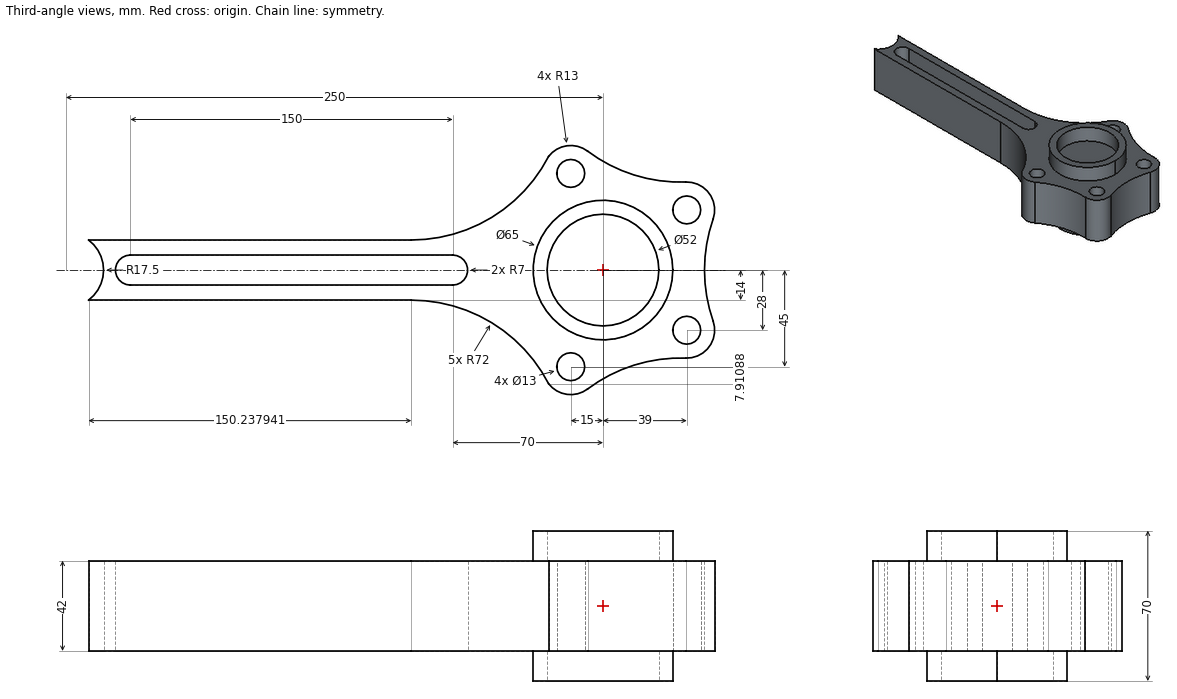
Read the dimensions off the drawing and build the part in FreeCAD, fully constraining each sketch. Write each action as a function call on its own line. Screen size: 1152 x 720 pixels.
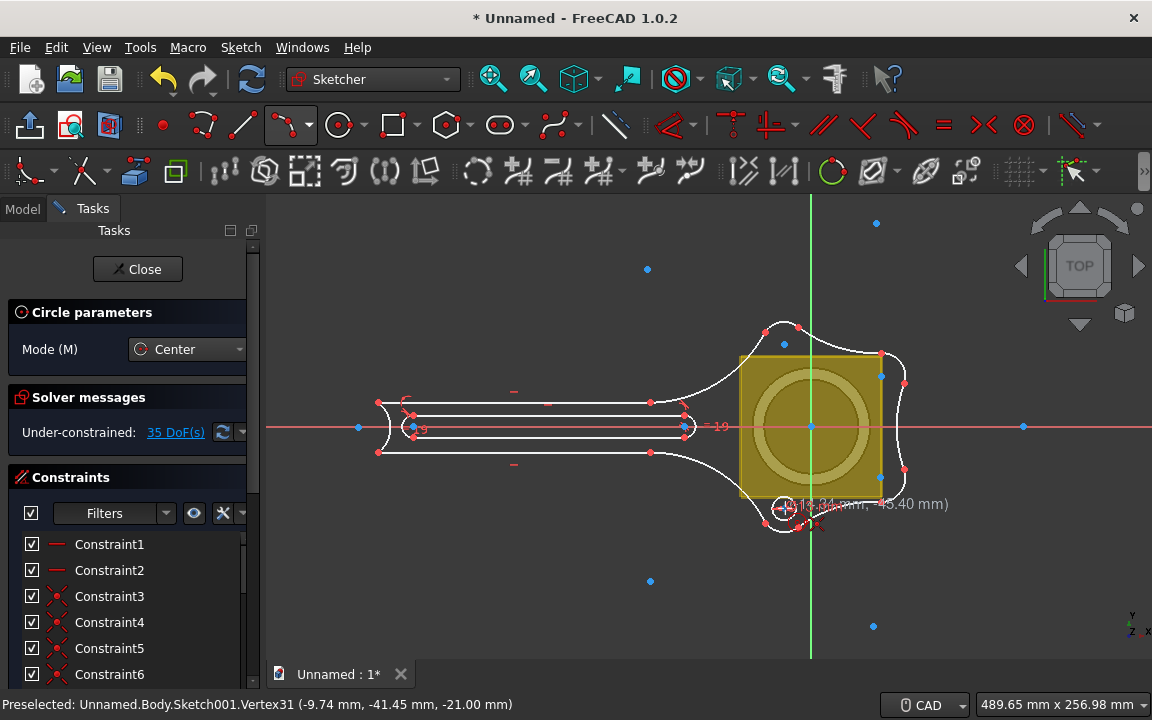
scroll(882, 477, up, 4)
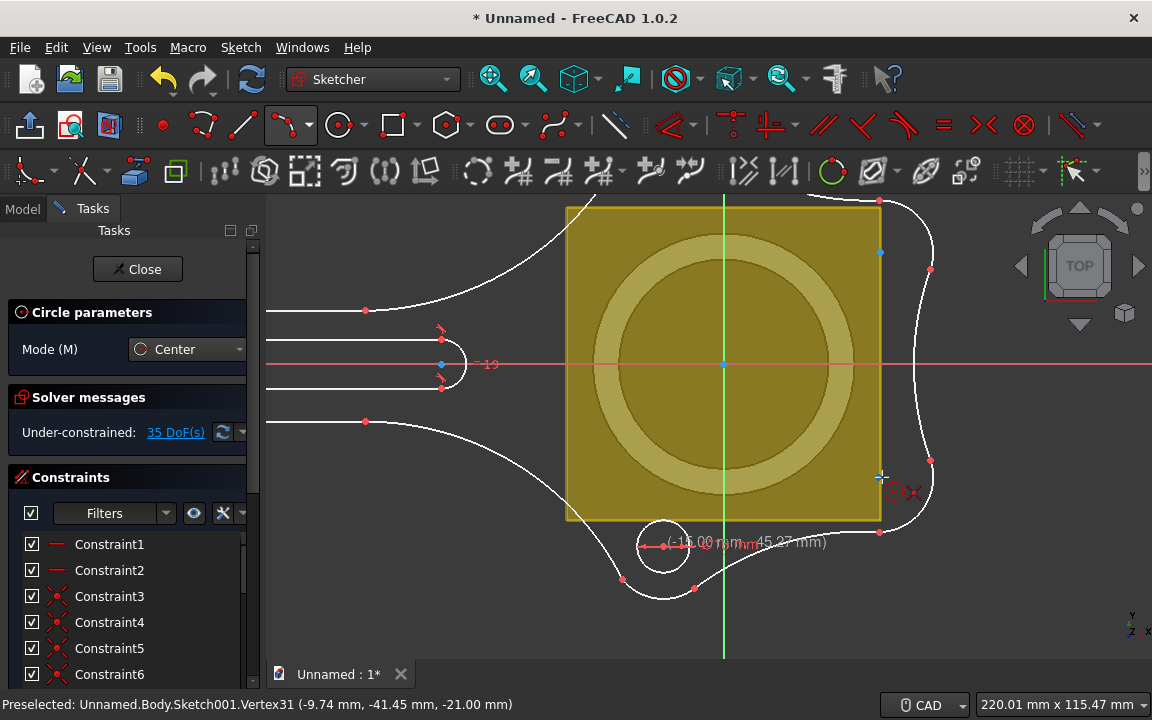
click(881, 477)
move(899, 458)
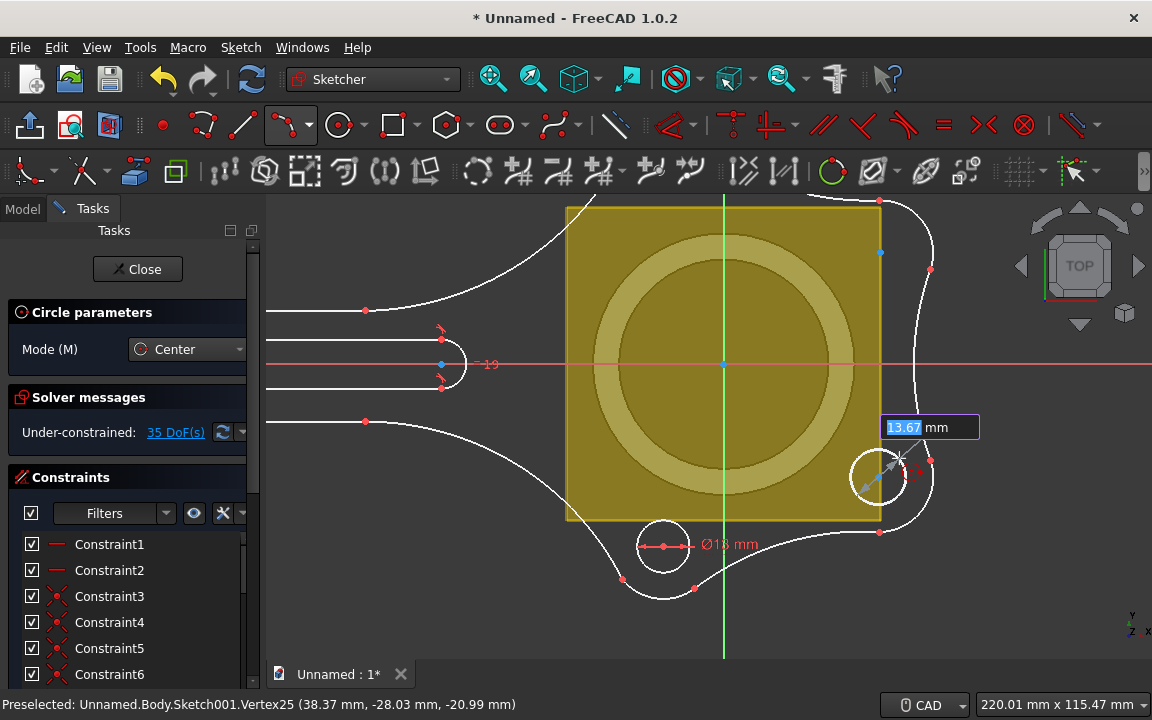
text(13)
key(Return)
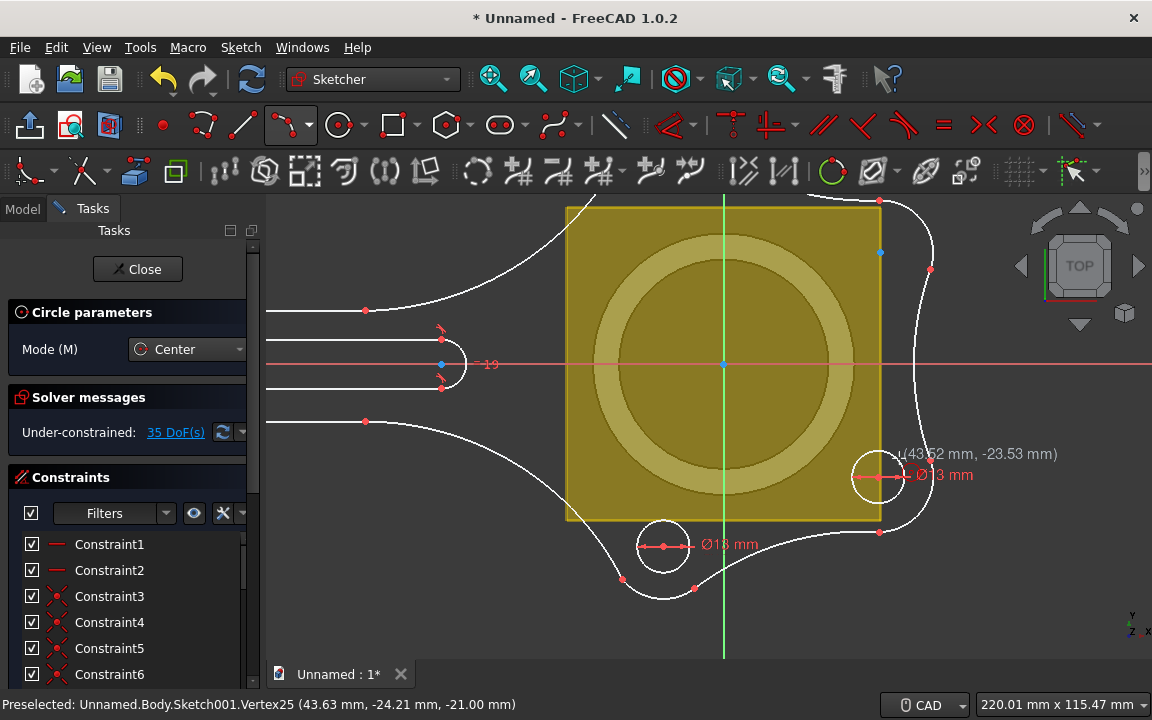
click(881, 251)
move(899, 233)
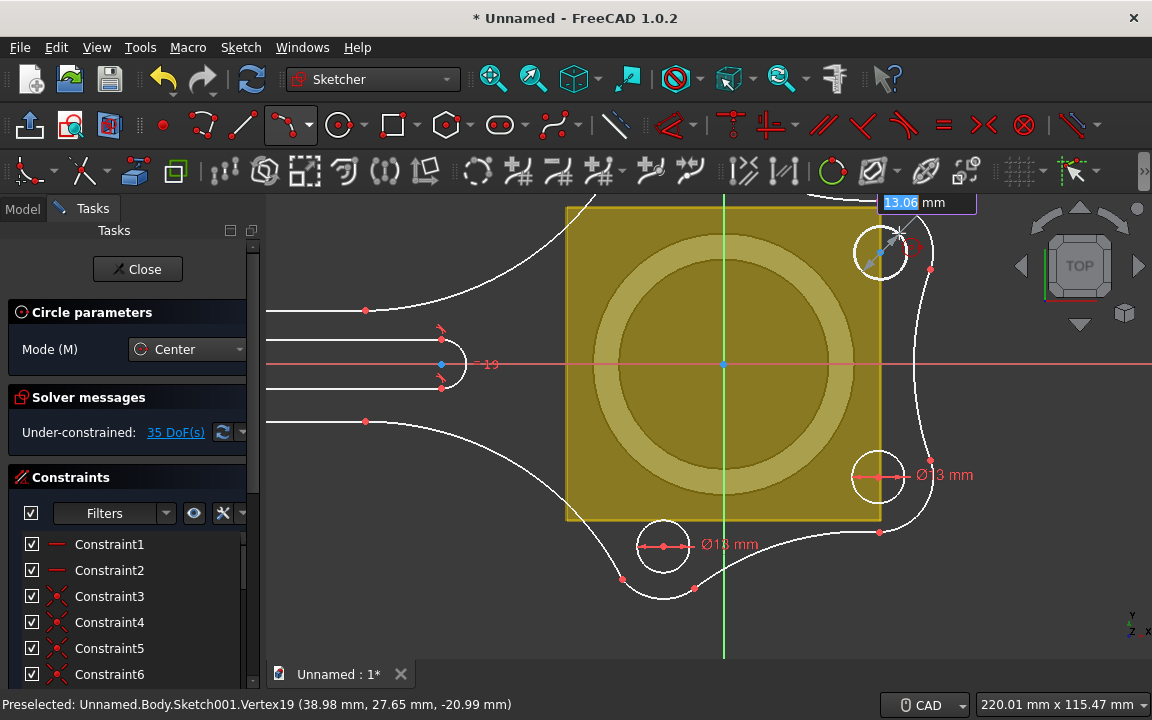
text(13)
key(Return)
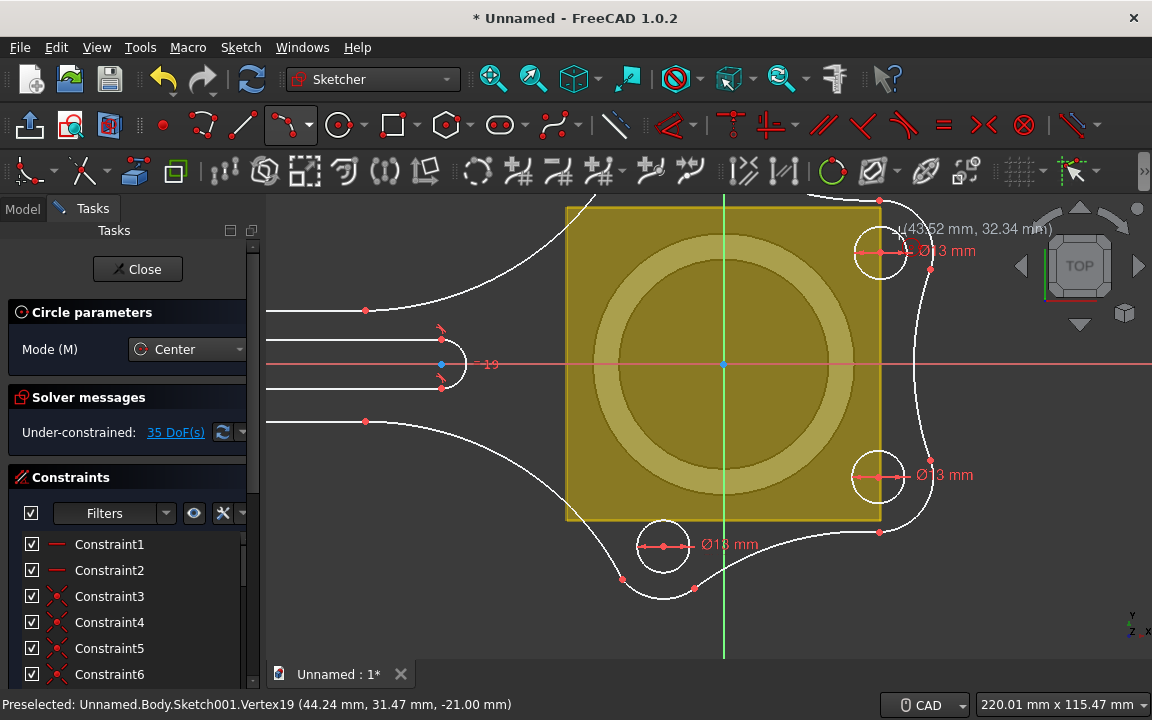
scroll(882, 477, down, 4)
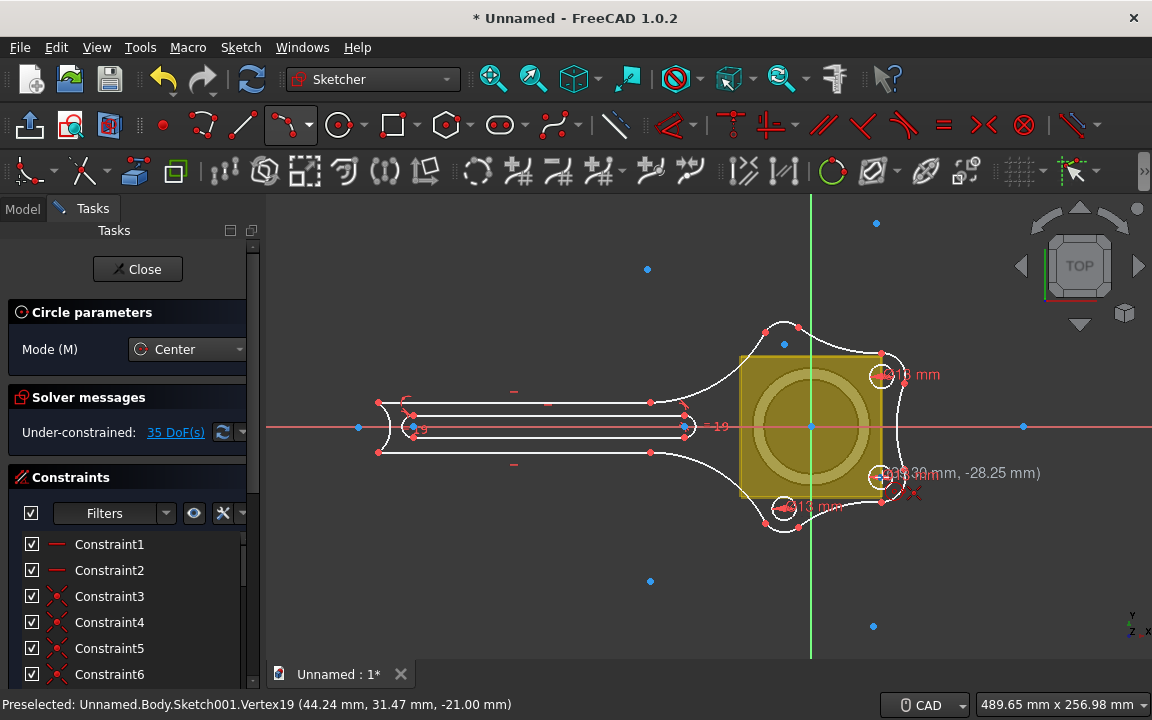
scroll(784, 345, up, 4)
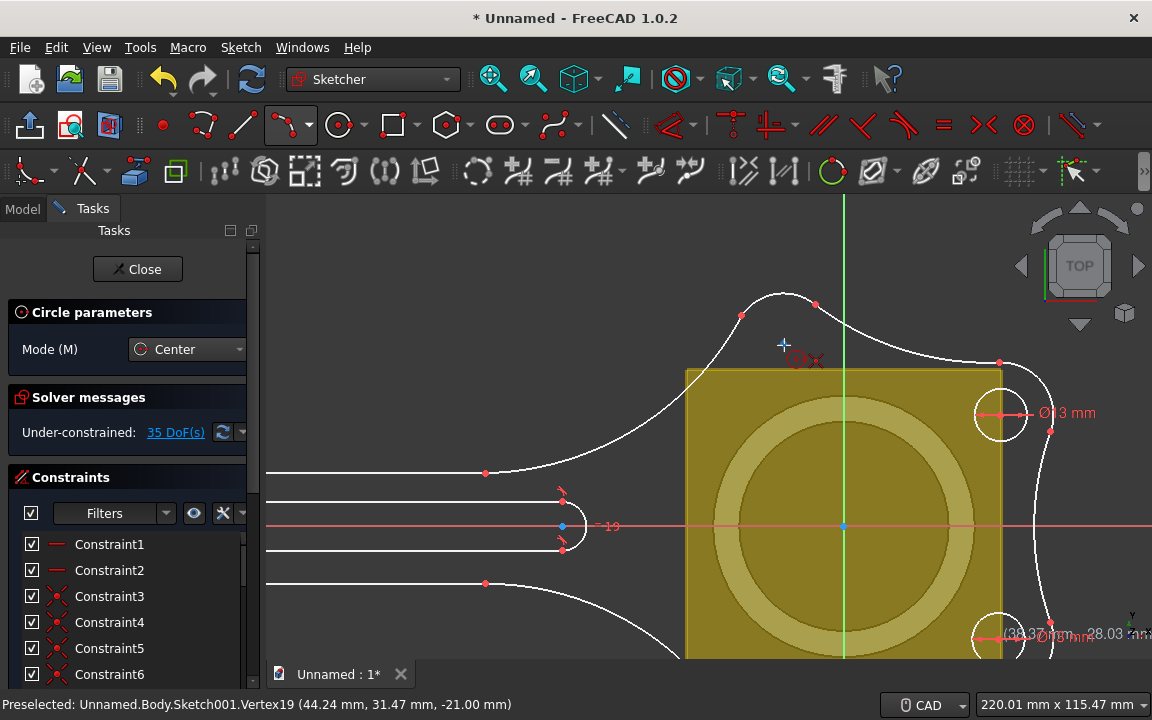
click(784, 345)
move(802, 327)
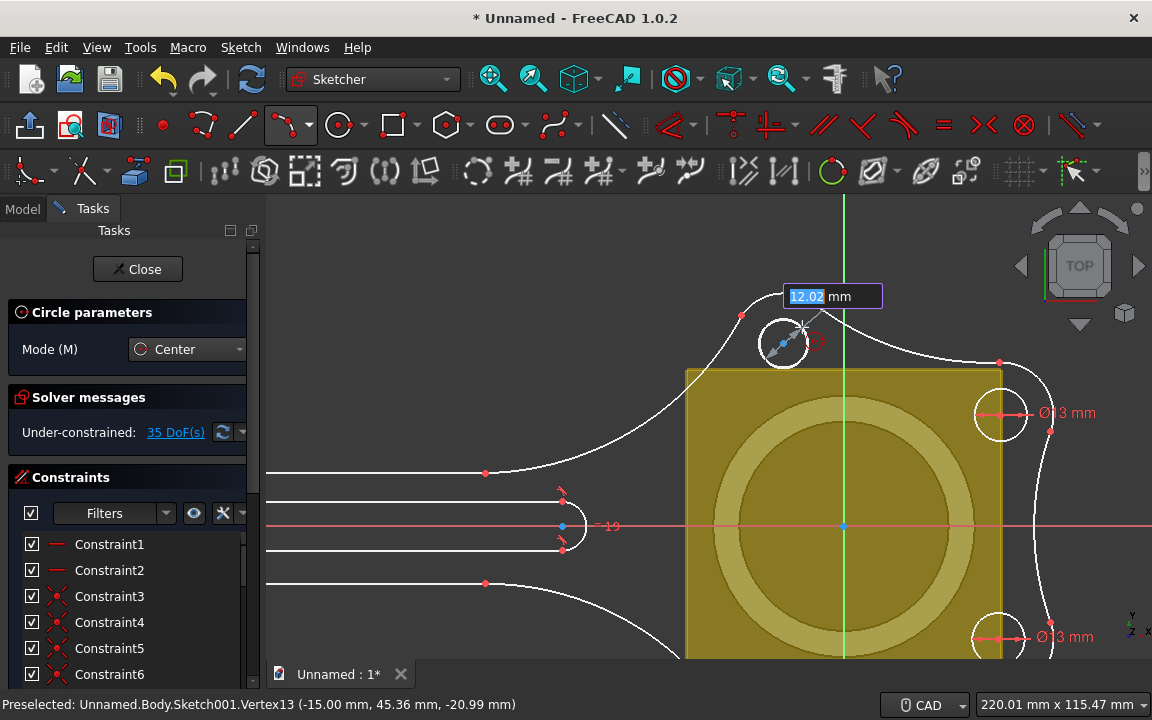
text(13)
key(Return)
key(Escape)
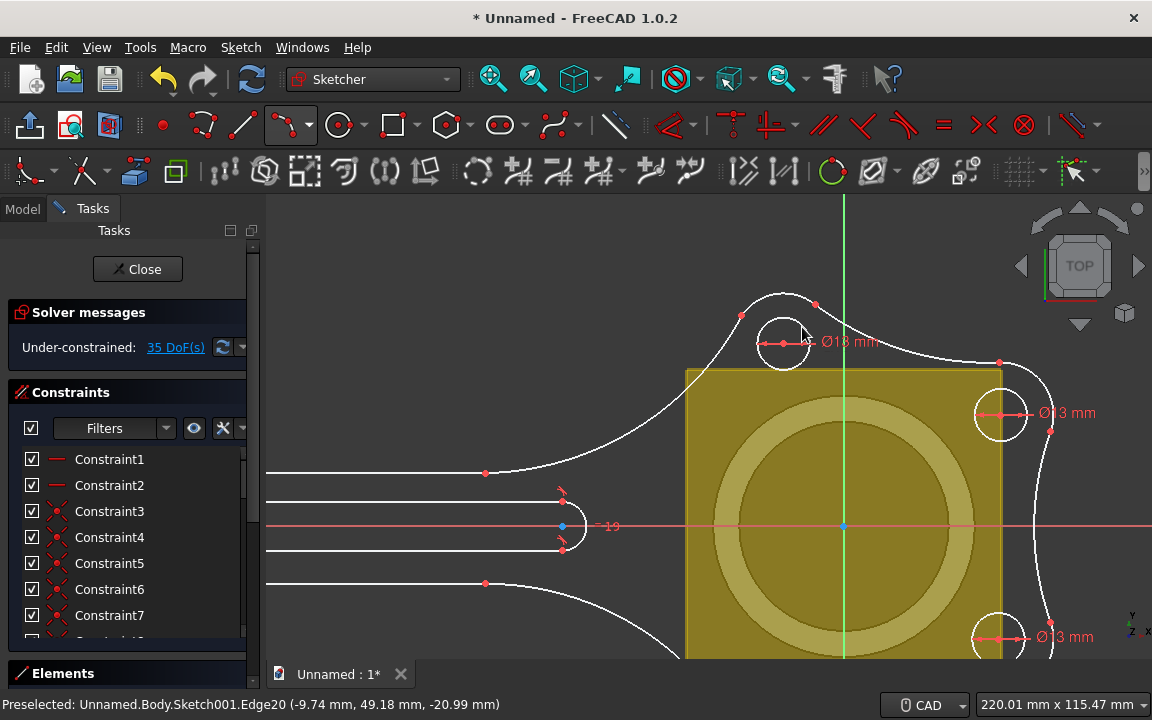
click(793, 294)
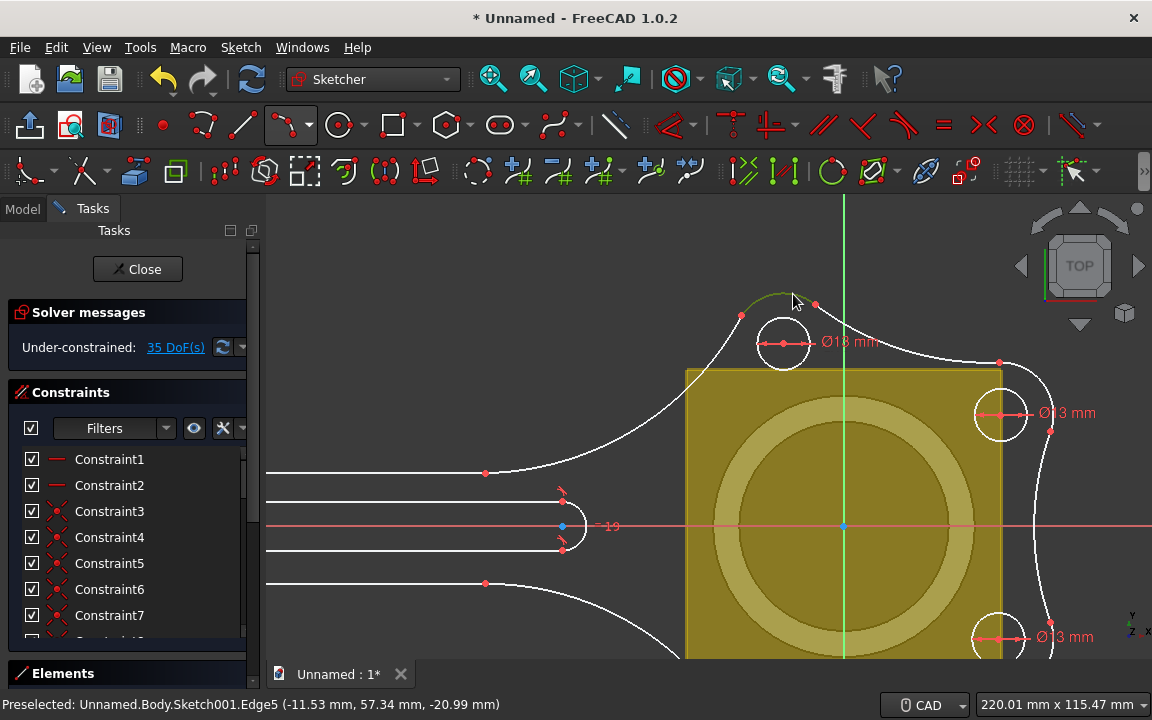
click(866, 335)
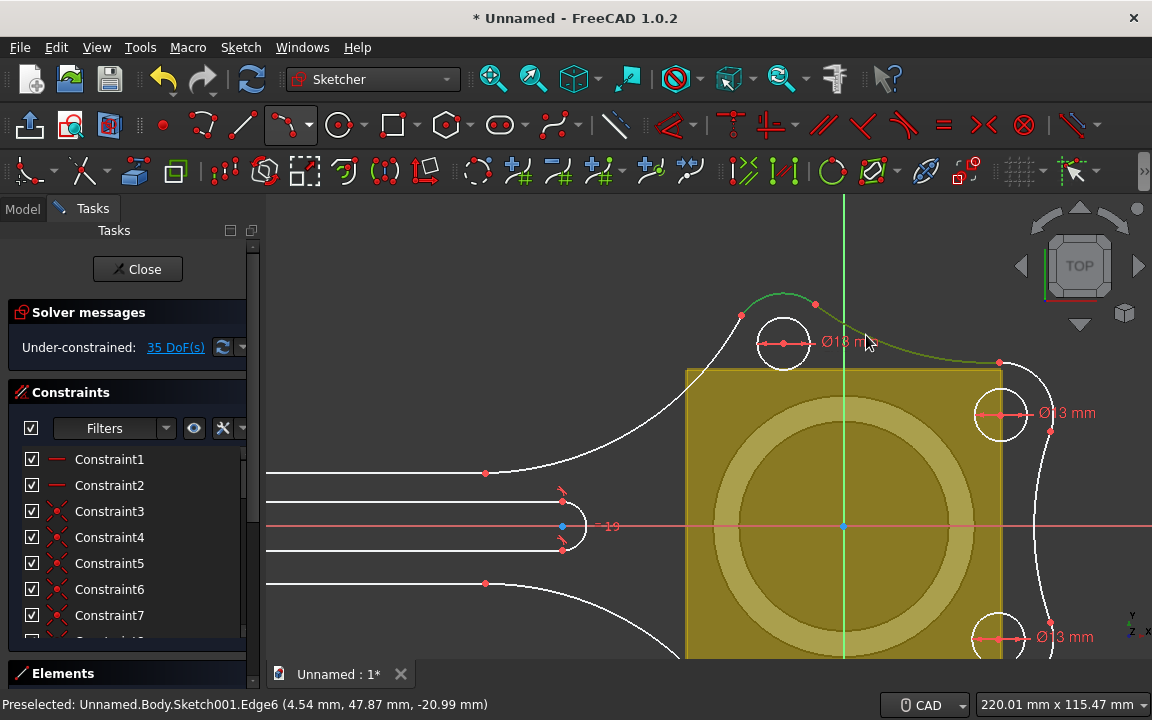
click(904, 126)